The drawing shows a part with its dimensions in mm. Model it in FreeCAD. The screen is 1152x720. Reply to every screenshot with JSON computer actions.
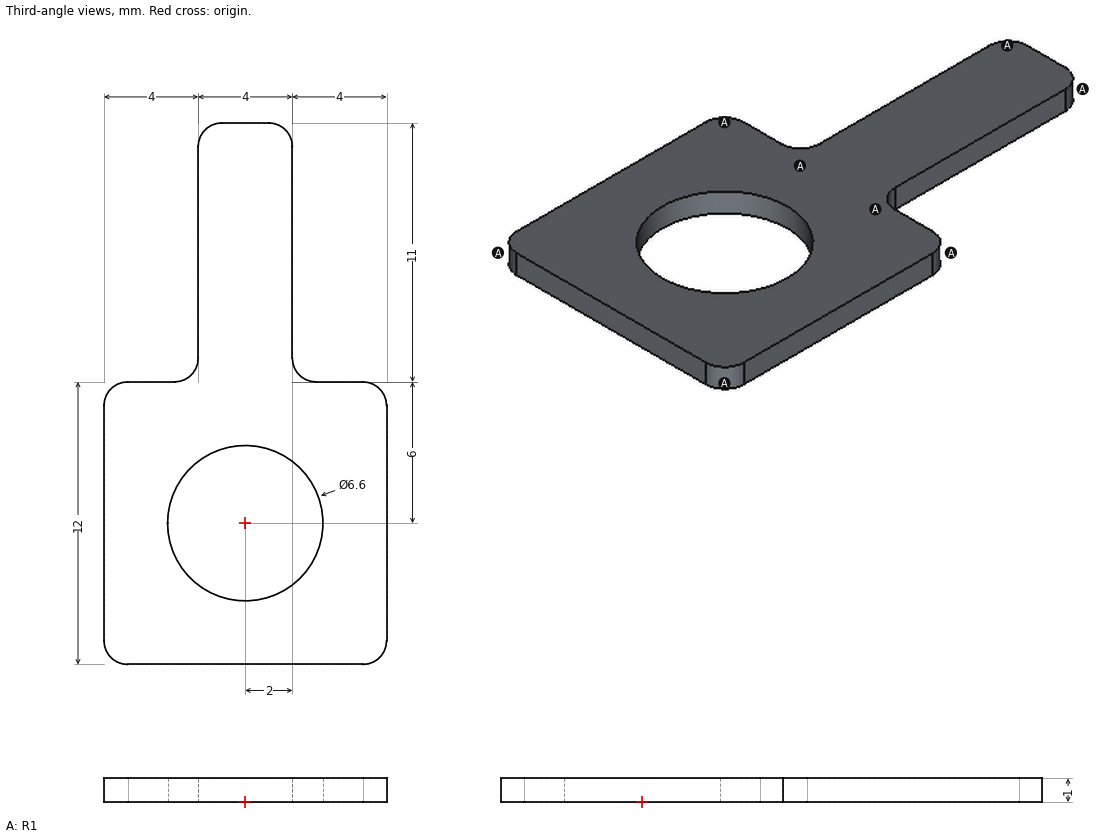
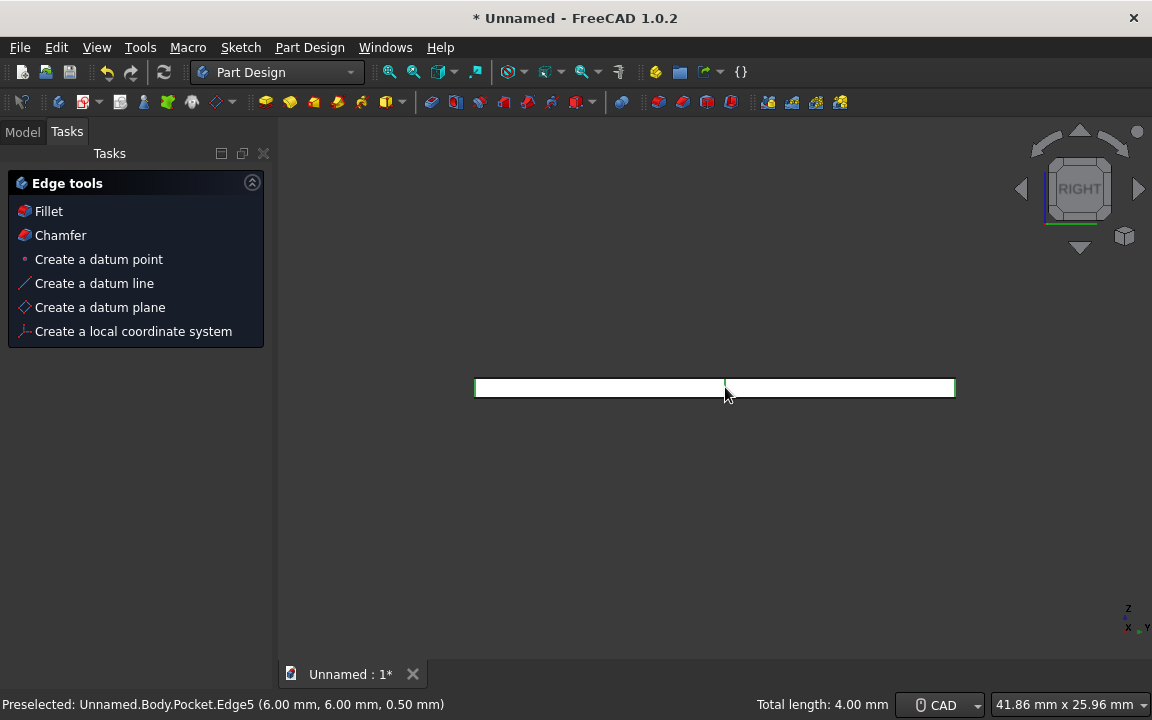
{"action": "key", "text": "5"}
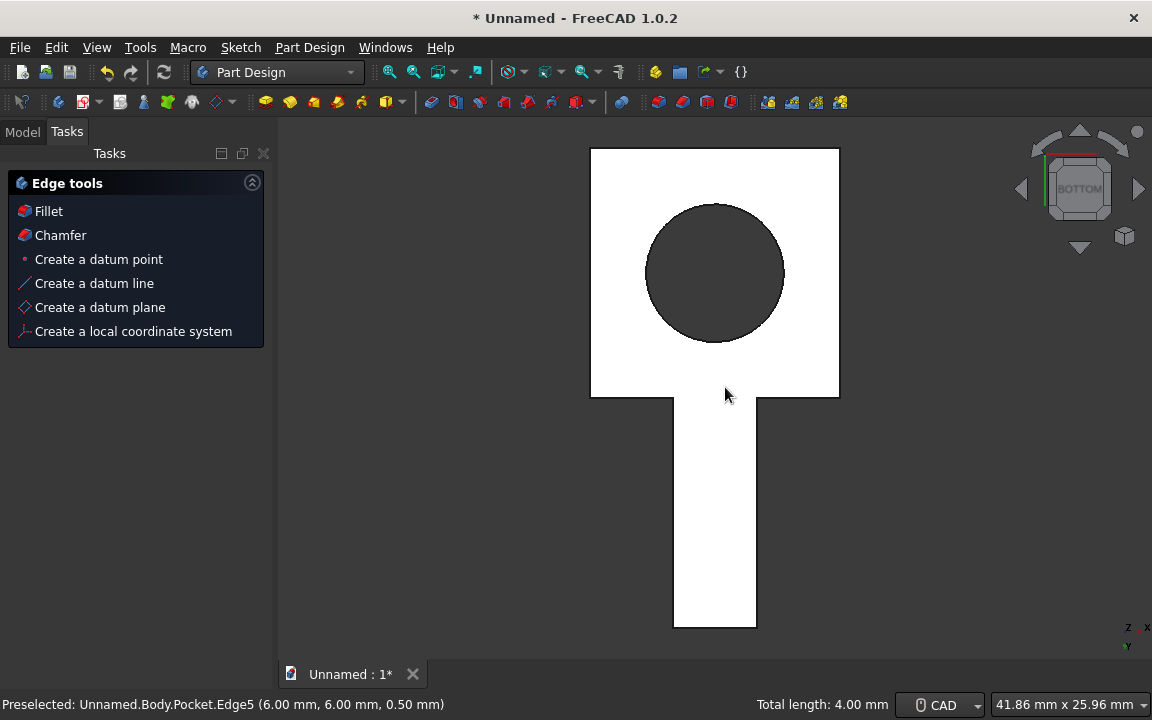
{"action": "scroll", "coordinate": [590, 397], "scroll_direction": "up", "scroll_amount": 4}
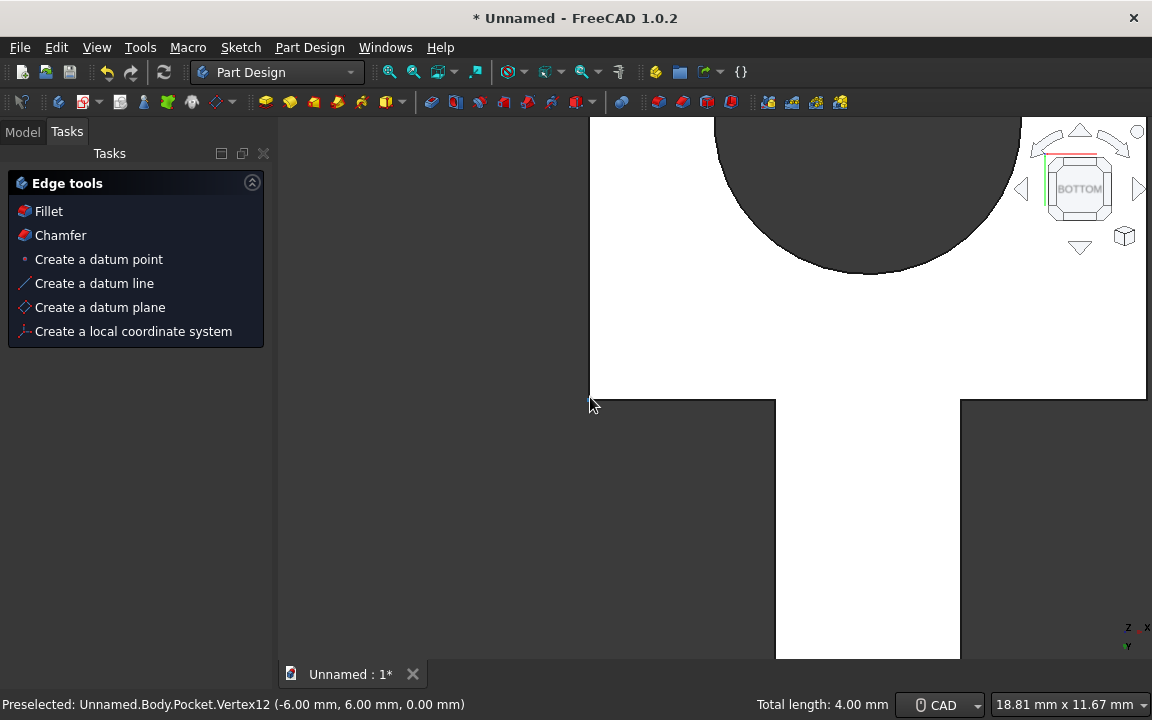
{"action": "key", "text": "v f"}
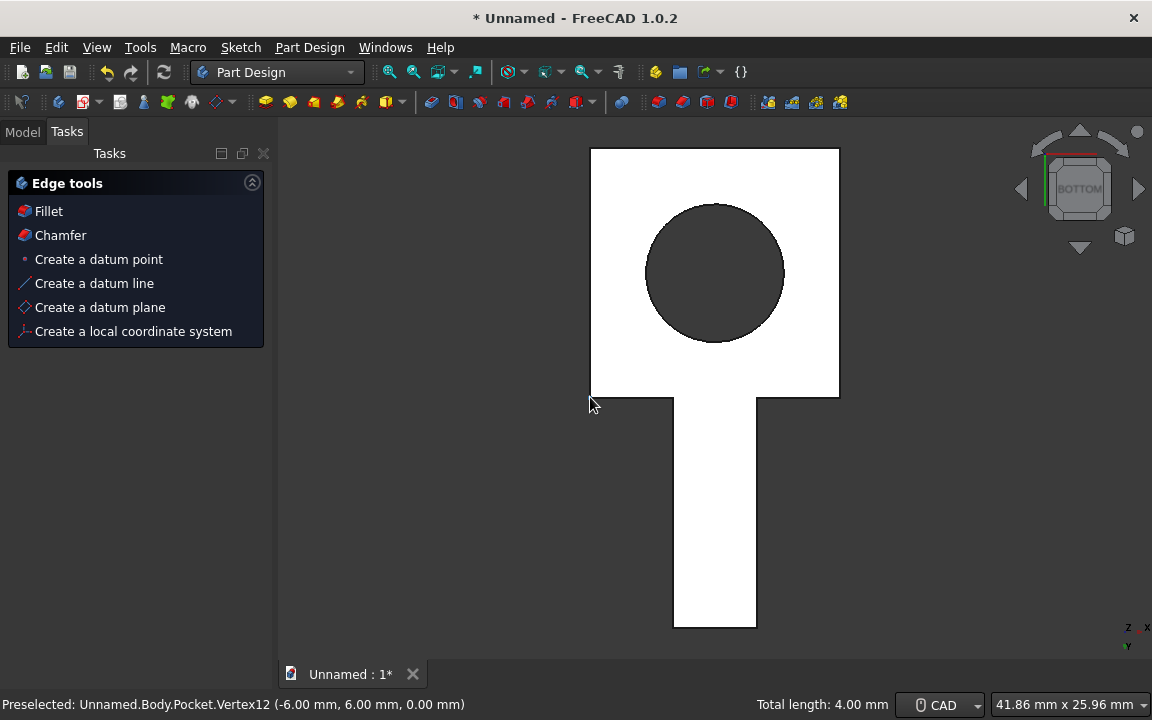
{"action": "key", "text": "4"}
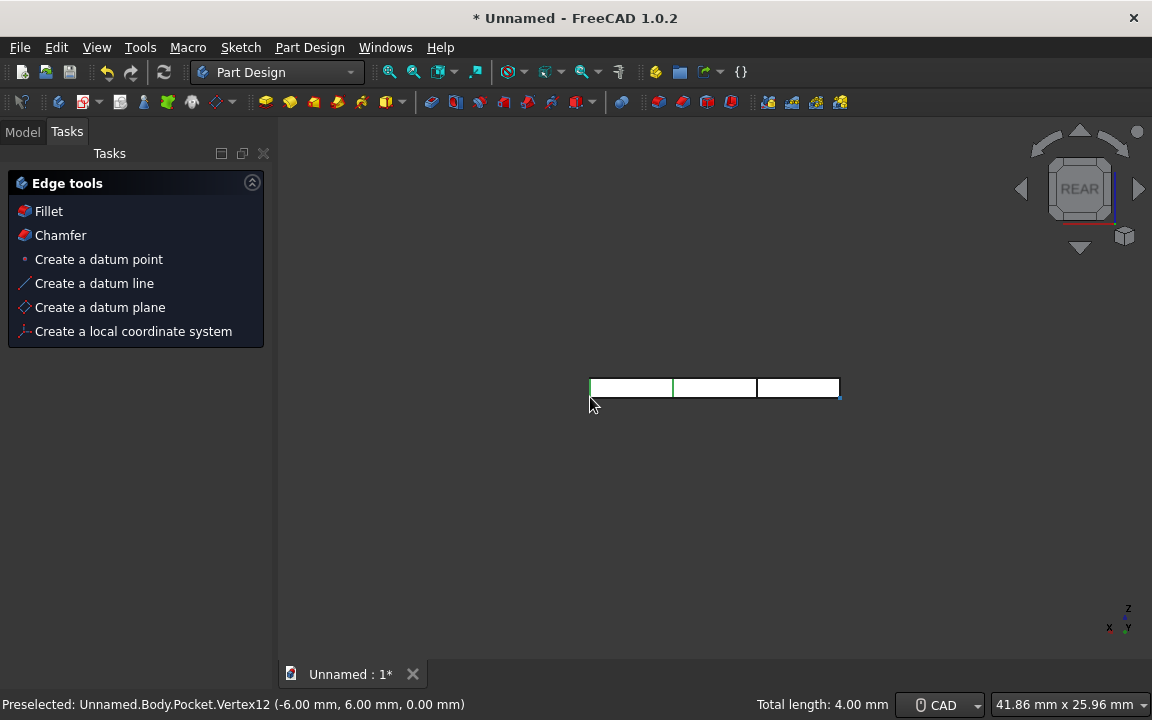
{"action": "key", "text": "v f"}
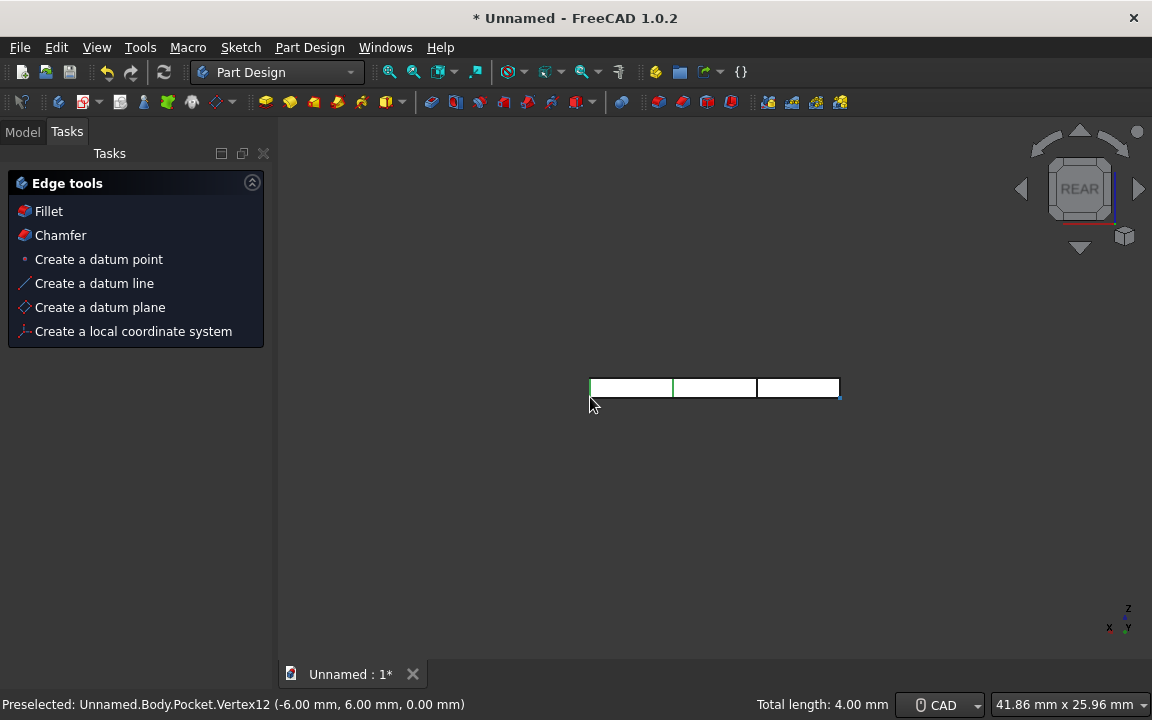
{"action": "left_click", "coordinate": [840, 387], "text": "ctrl"}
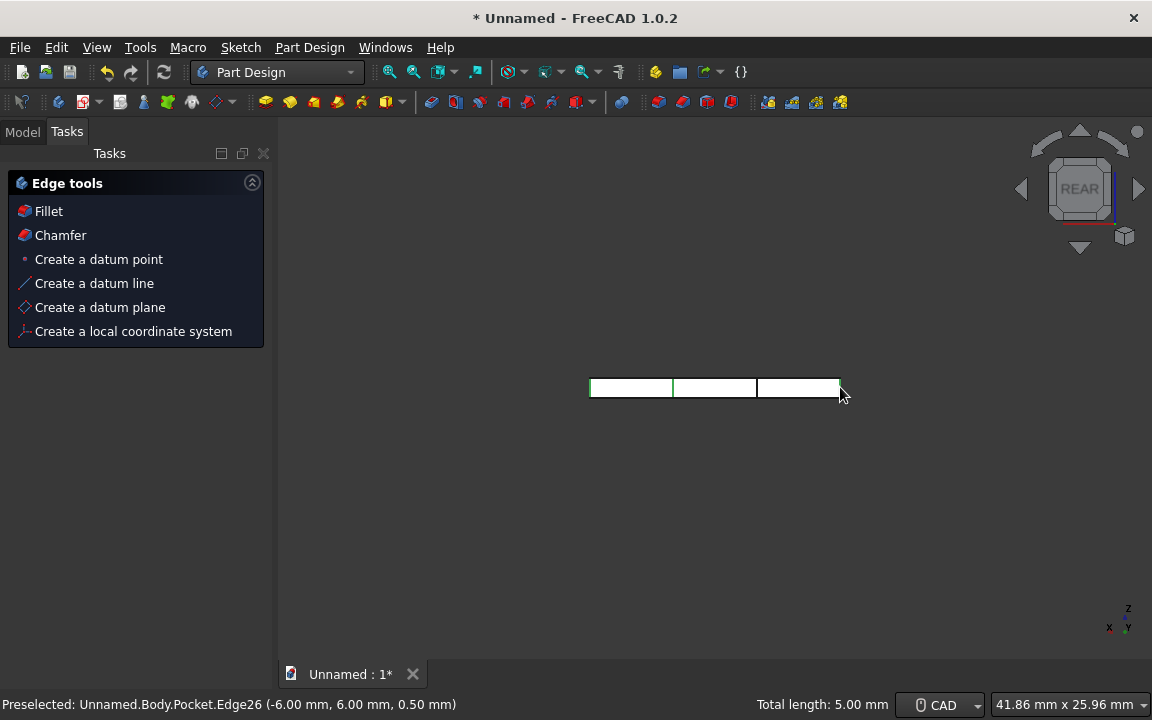
{"action": "left_click", "coordinate": [757, 387], "text": "ctrl"}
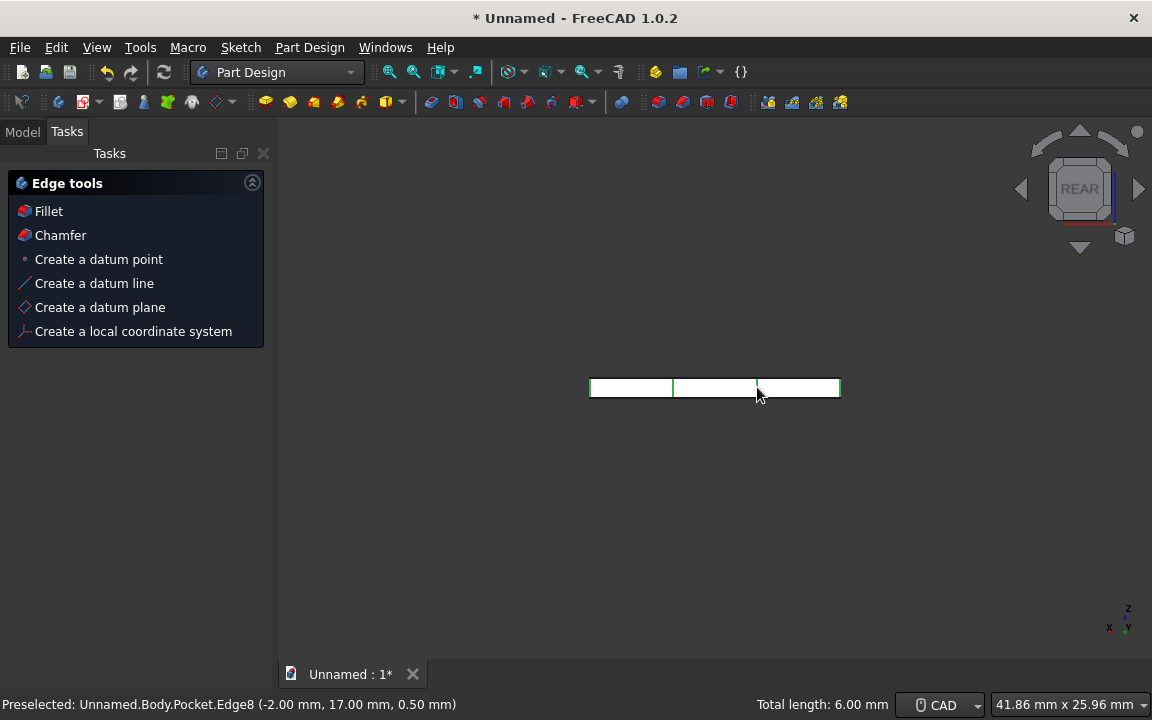
{"action": "scroll", "coordinate": [757, 387], "scroll_direction": "up", "scroll_amount": 4}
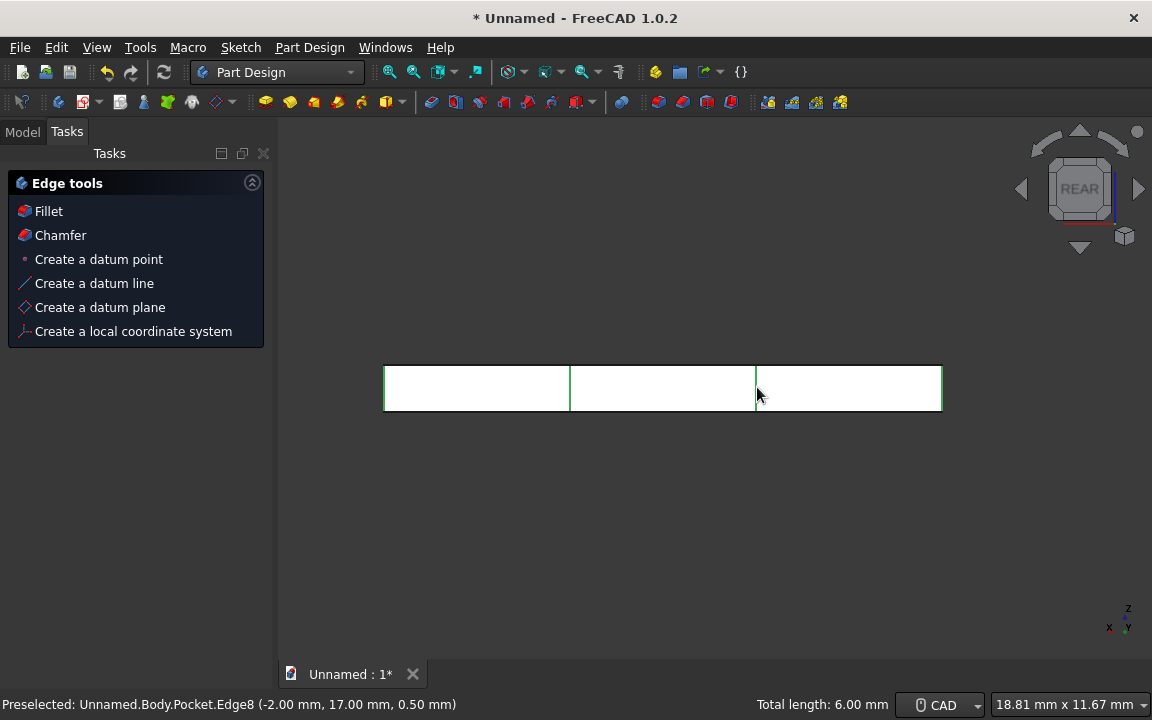
{"action": "key", "text": "v f"}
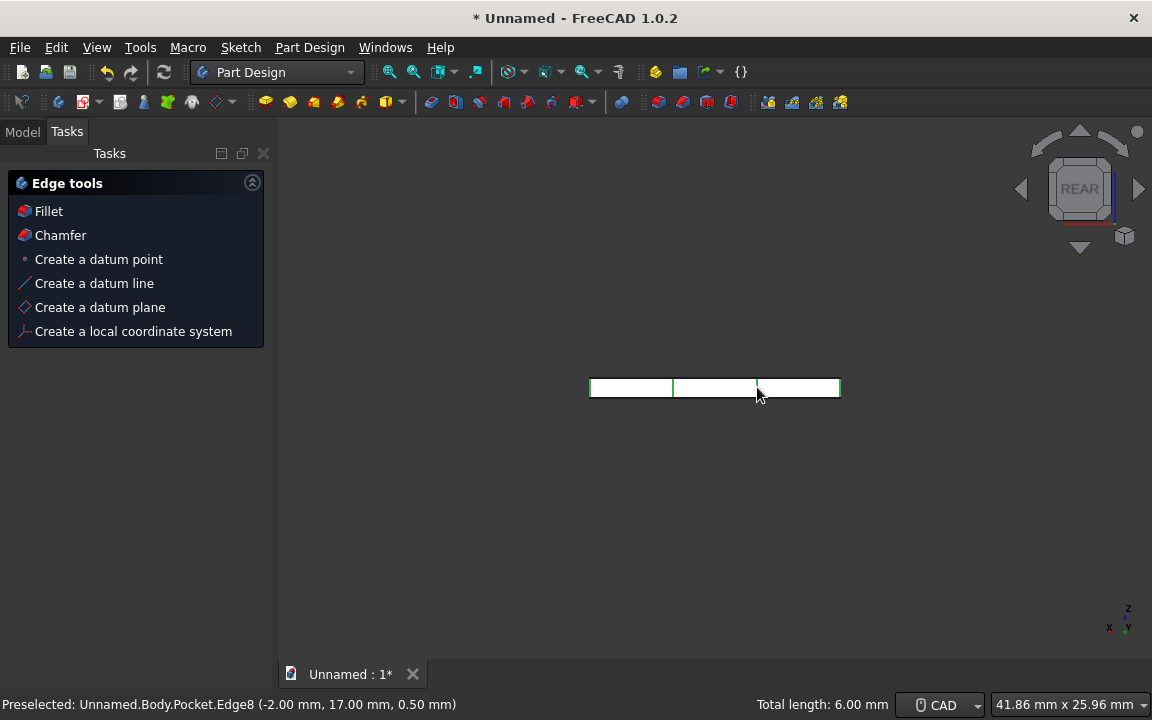
{"action": "key", "text": "6"}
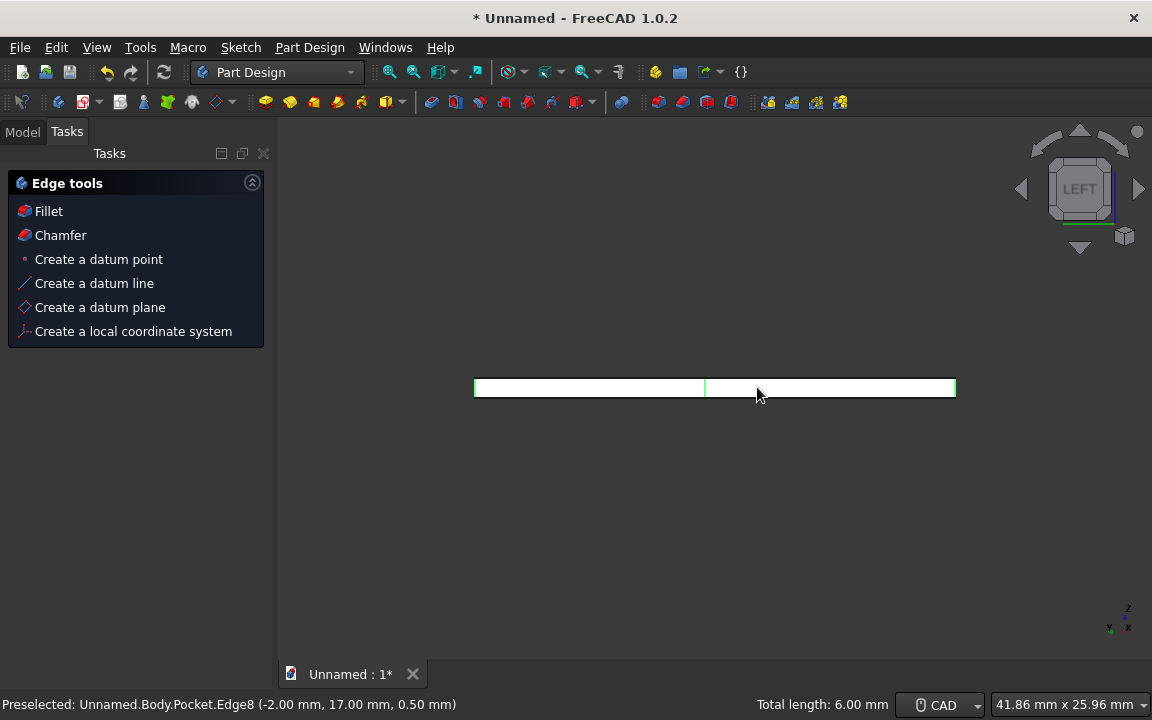
{"action": "scroll", "coordinate": [705, 387], "scroll_direction": "up", "scroll_amount": 4}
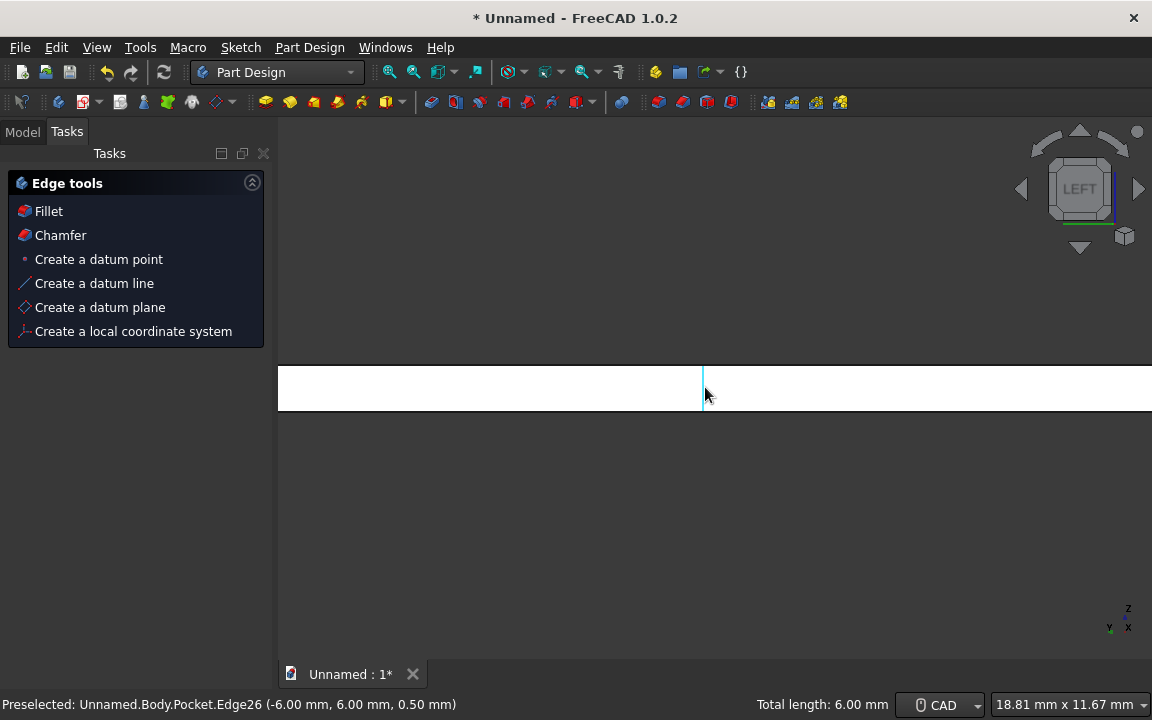
{"action": "key", "text": "v f"}